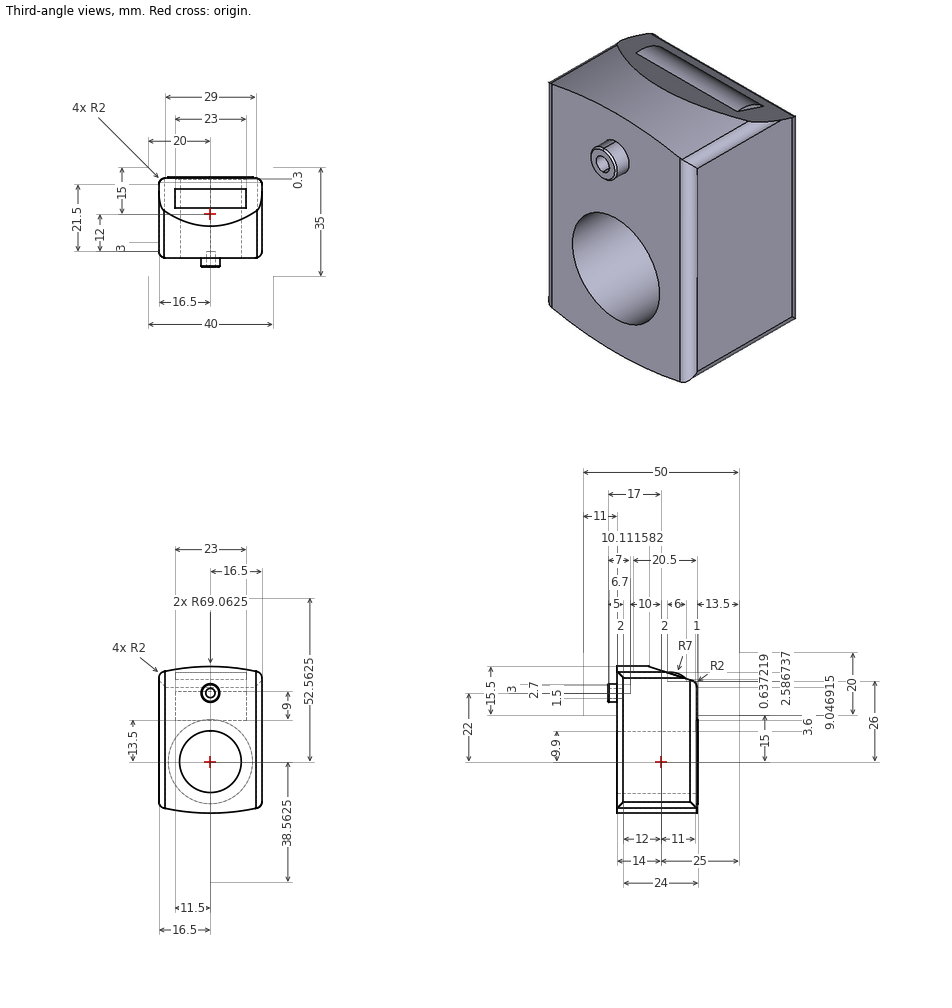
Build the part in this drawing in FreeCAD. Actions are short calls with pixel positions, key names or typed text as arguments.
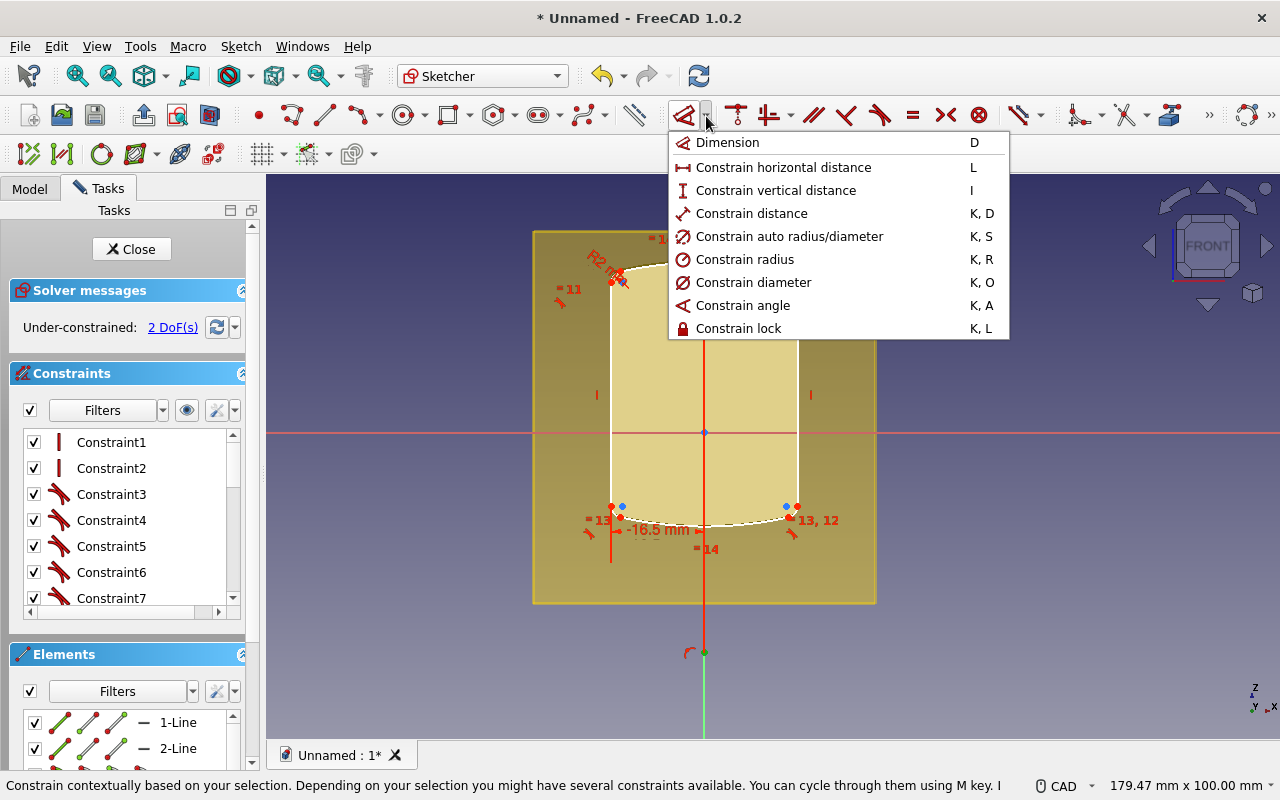
click(839, 190)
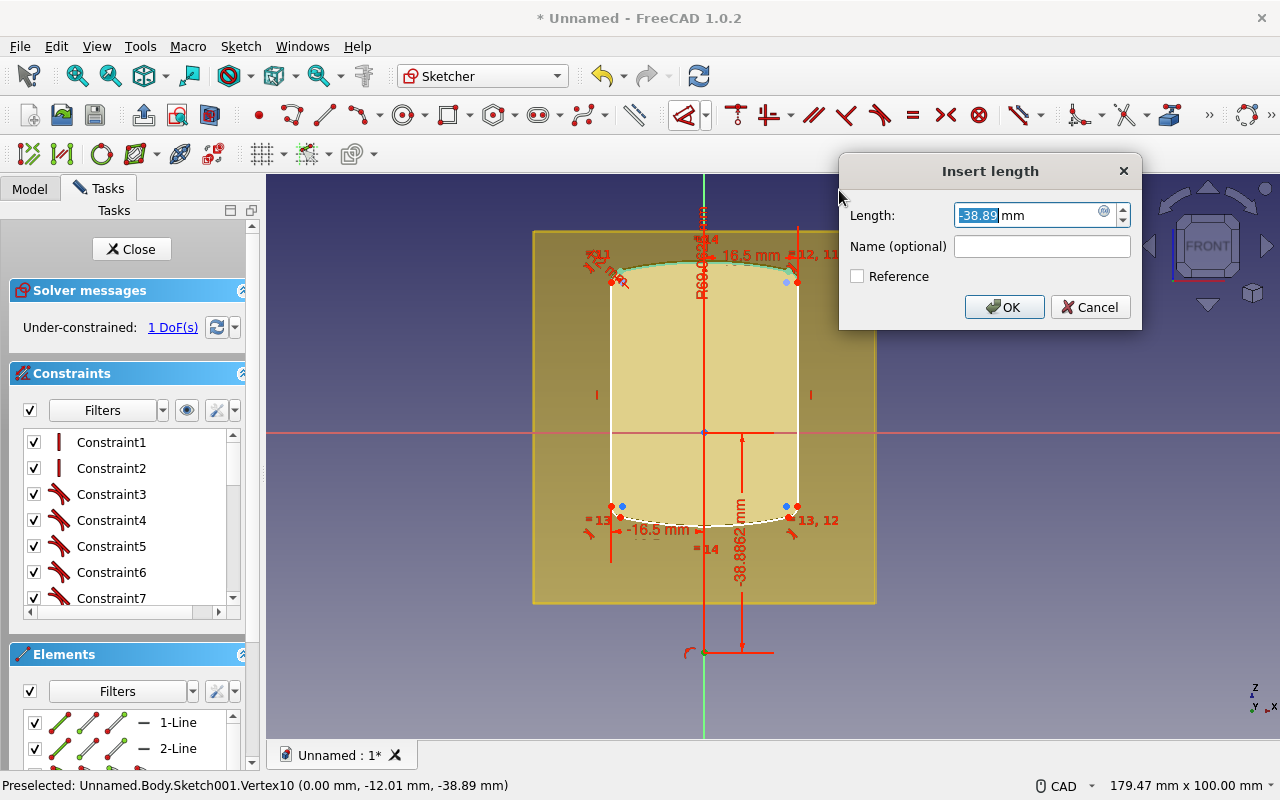
text(-38.5625)
key(Return)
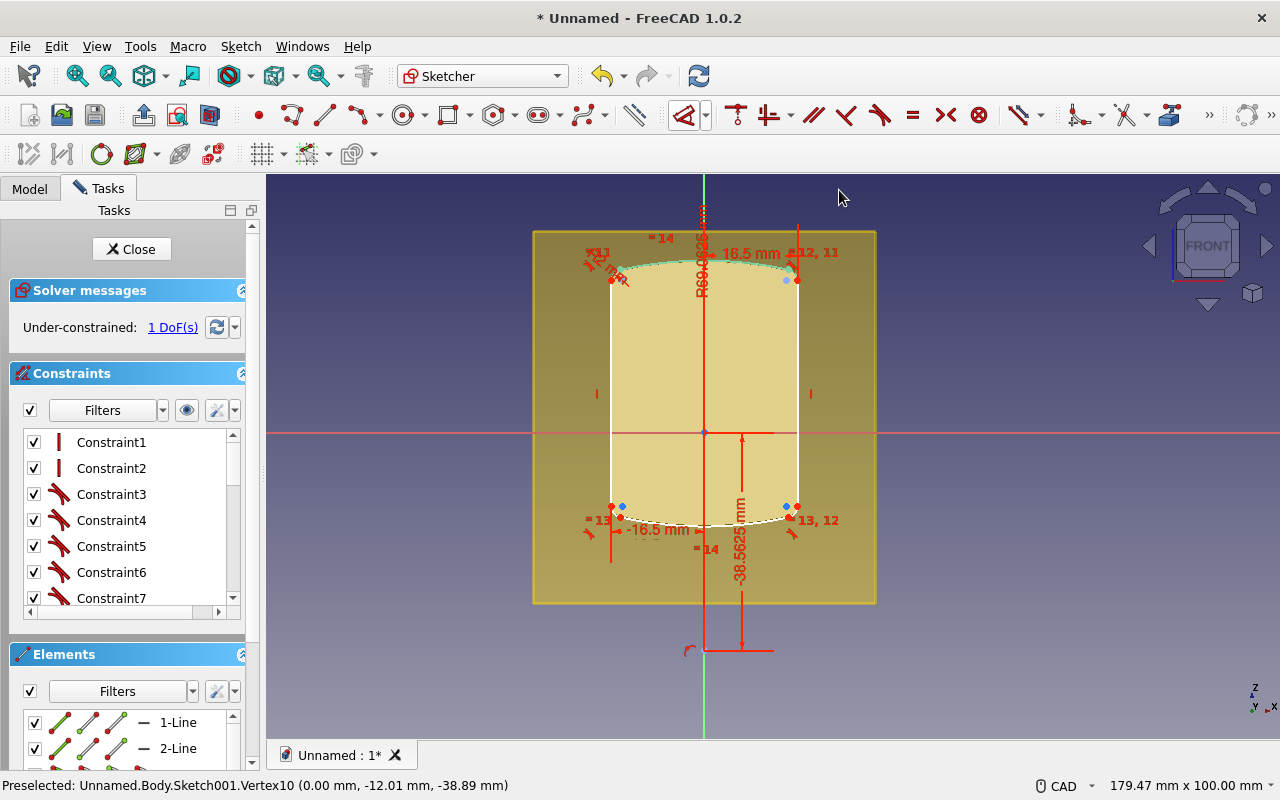
scroll(704, 265, up, 2)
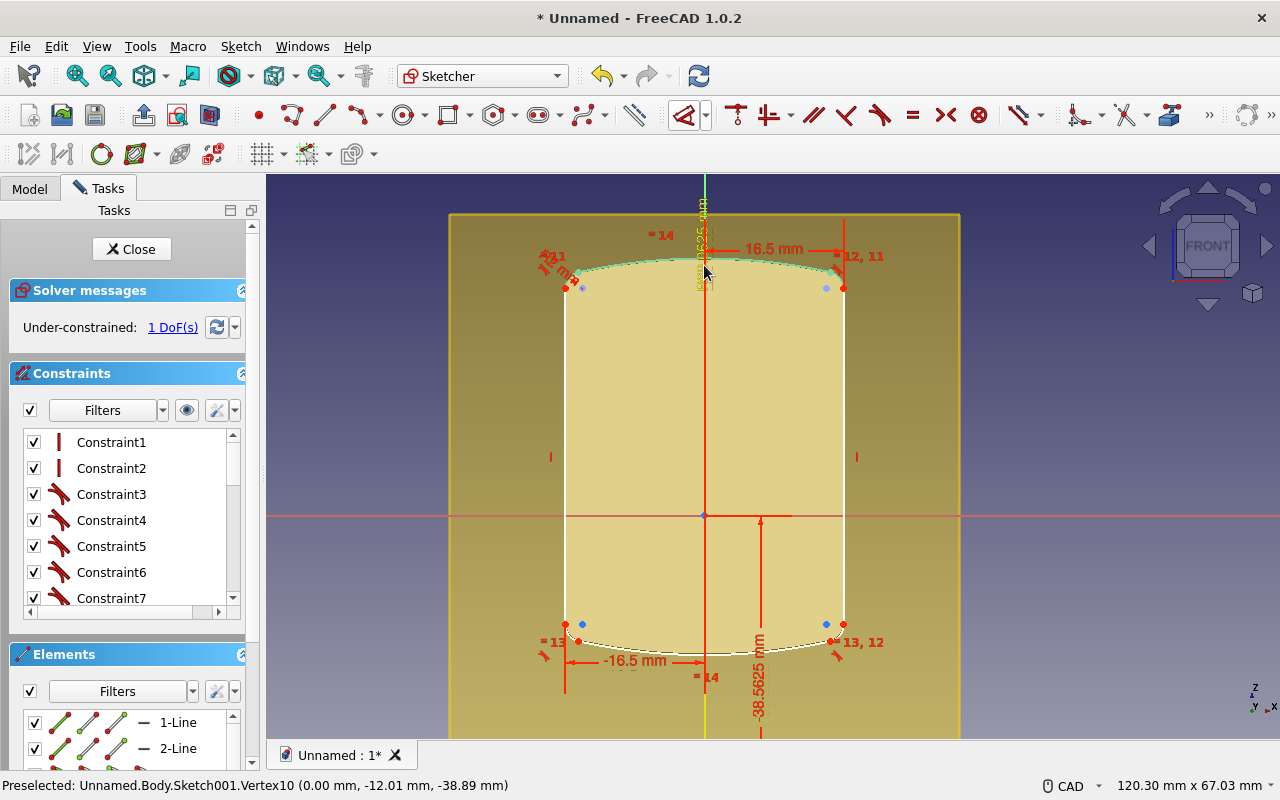
scroll(704, 645, down, 2)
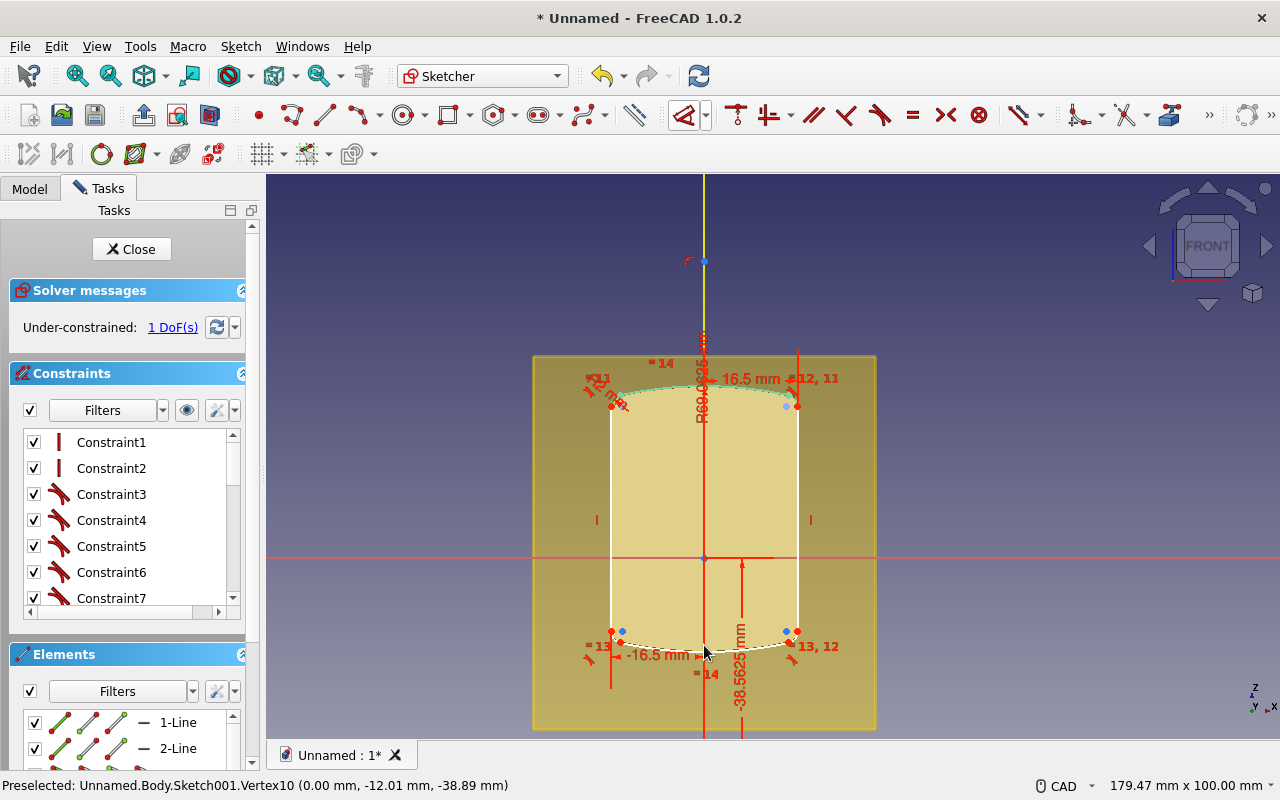
click(704, 262)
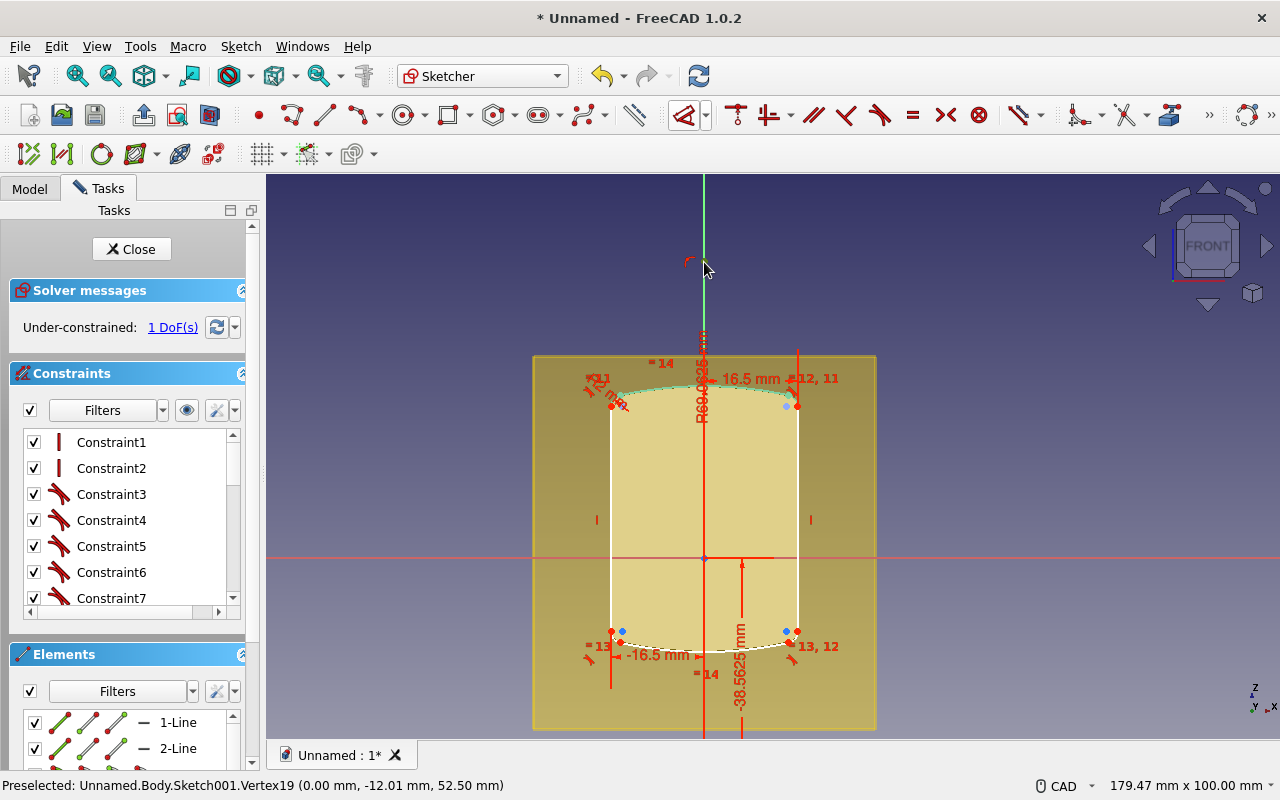
key(i)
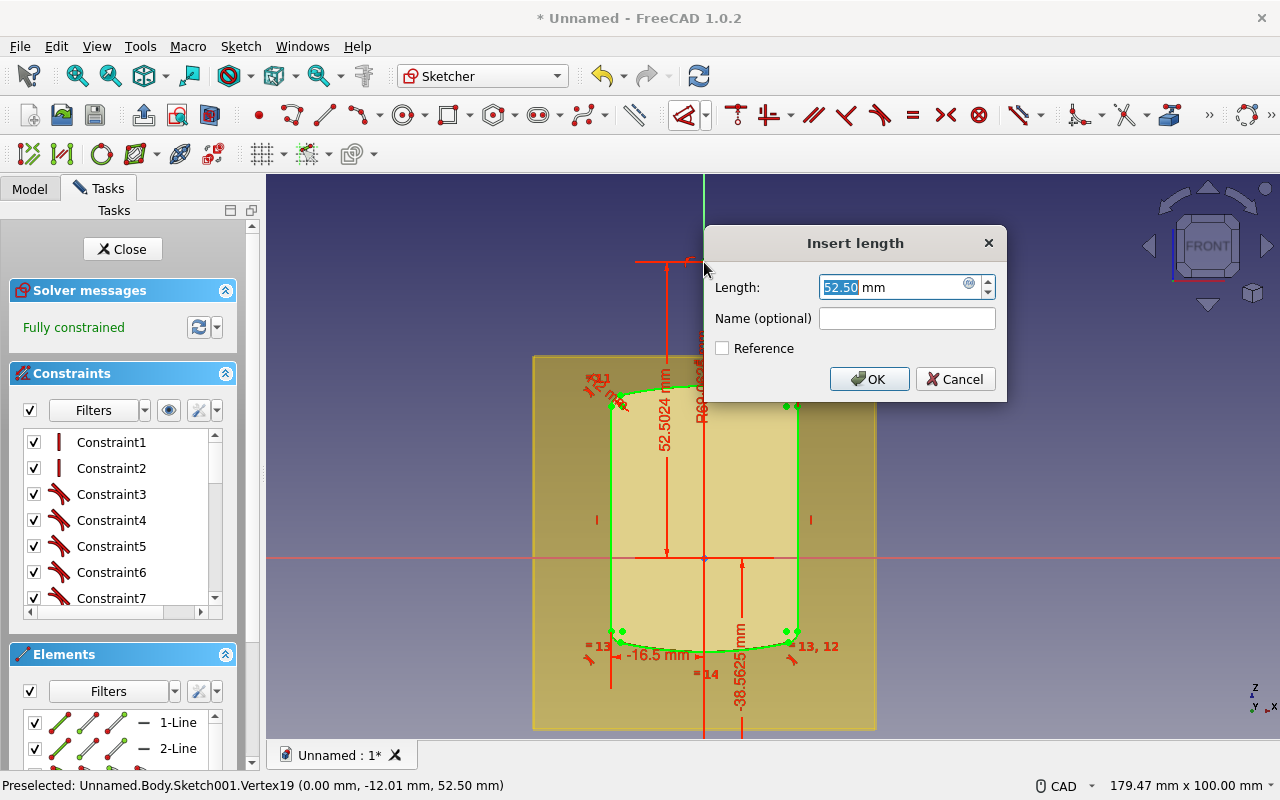
text(52.5625)
key(Return)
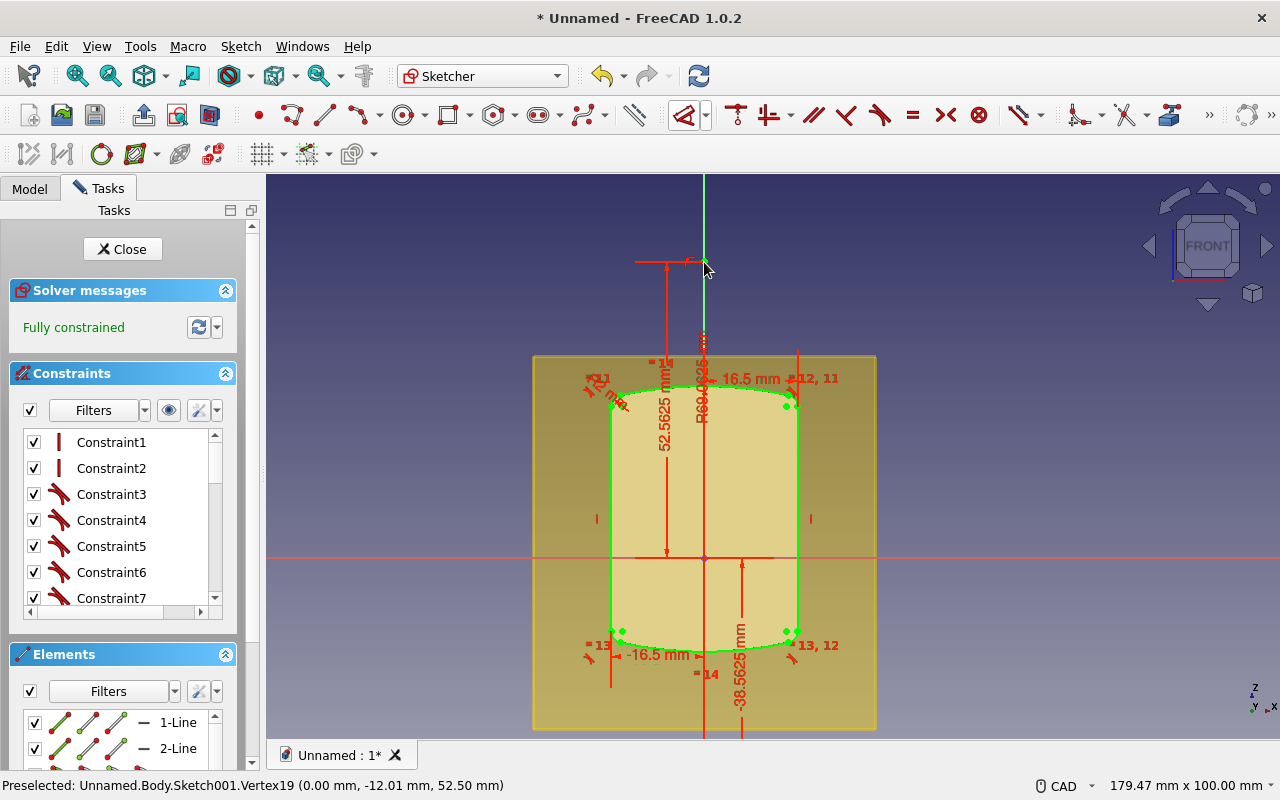
click(123, 249)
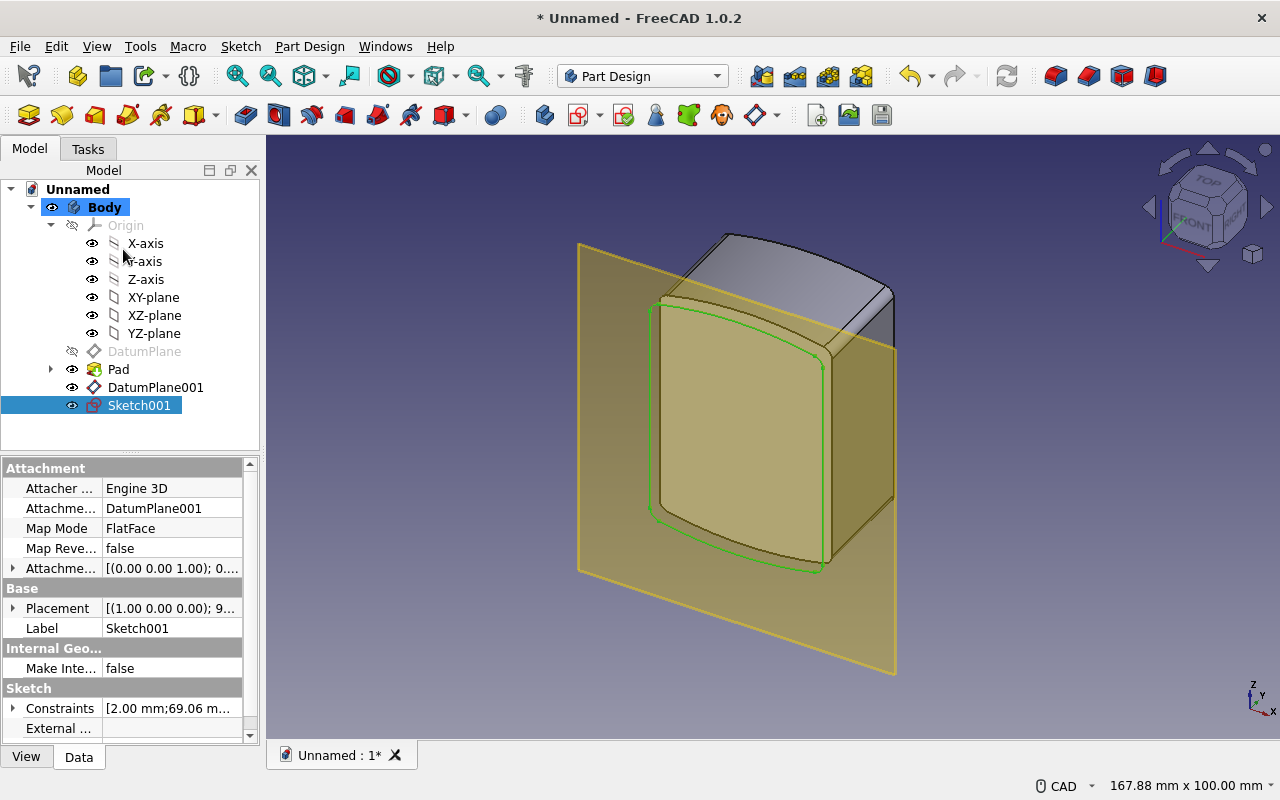
click(29, 116)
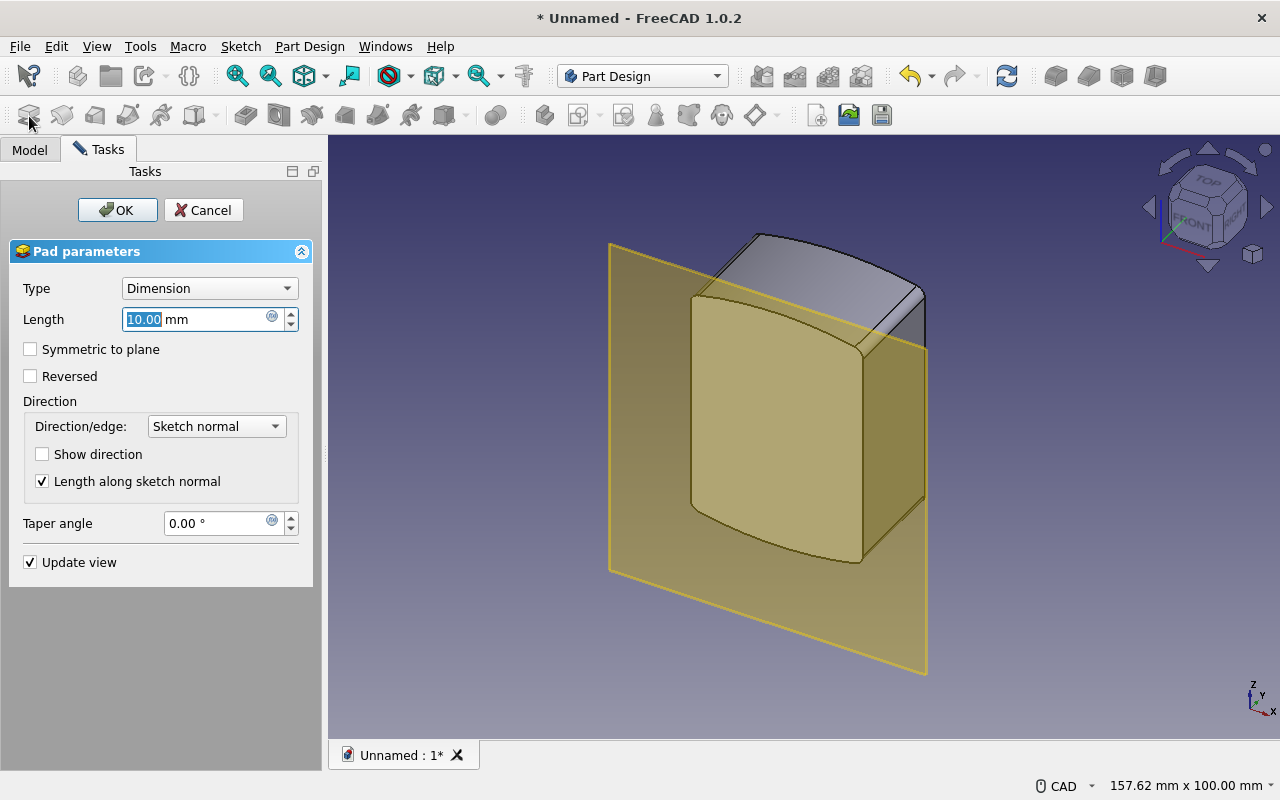
text(3)
key(Tab)